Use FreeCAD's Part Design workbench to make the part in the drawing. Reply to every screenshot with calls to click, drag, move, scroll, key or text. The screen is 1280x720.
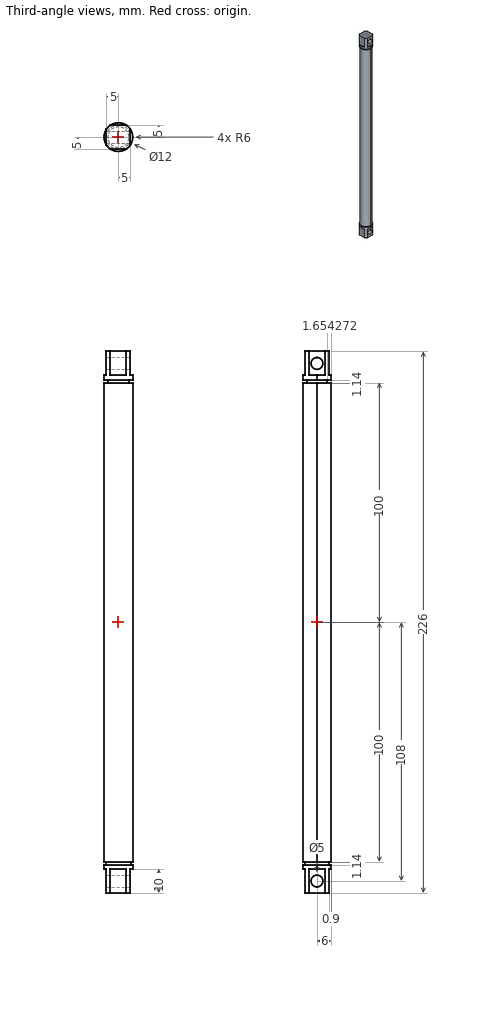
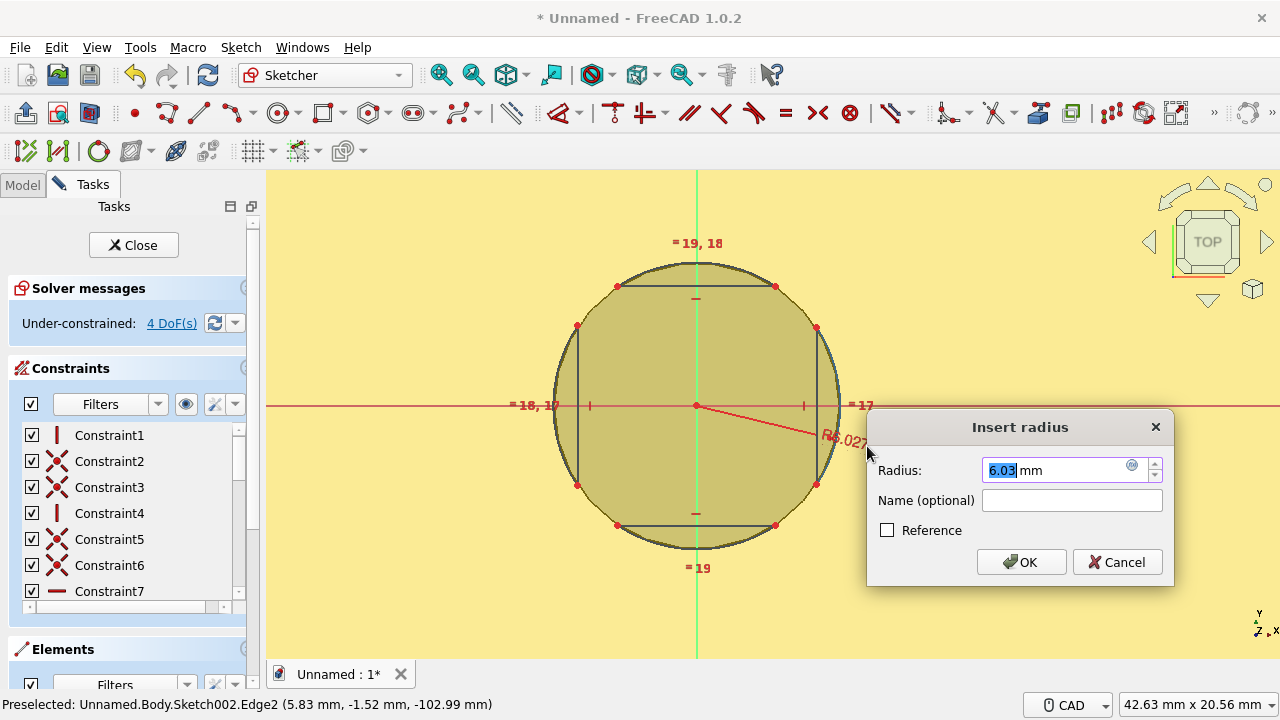
text(6)
key(Return)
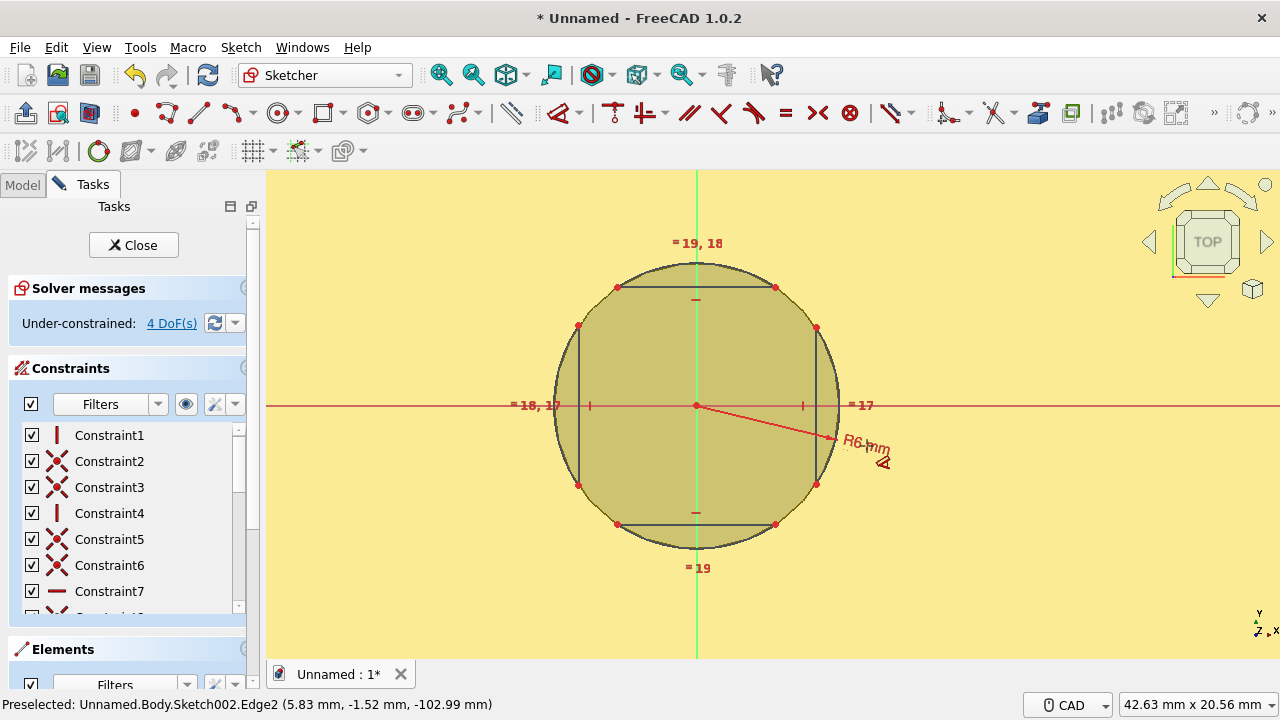
click(816, 484)
click(798, 518)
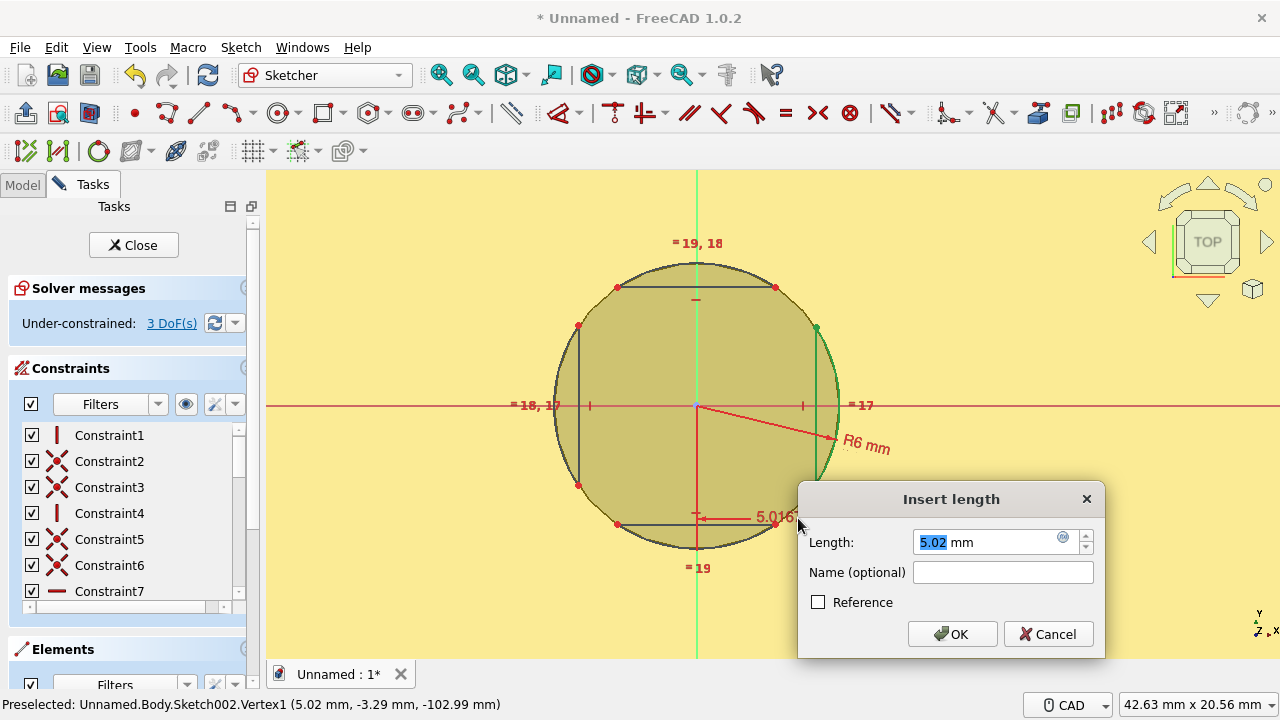
text(5)
key(Return)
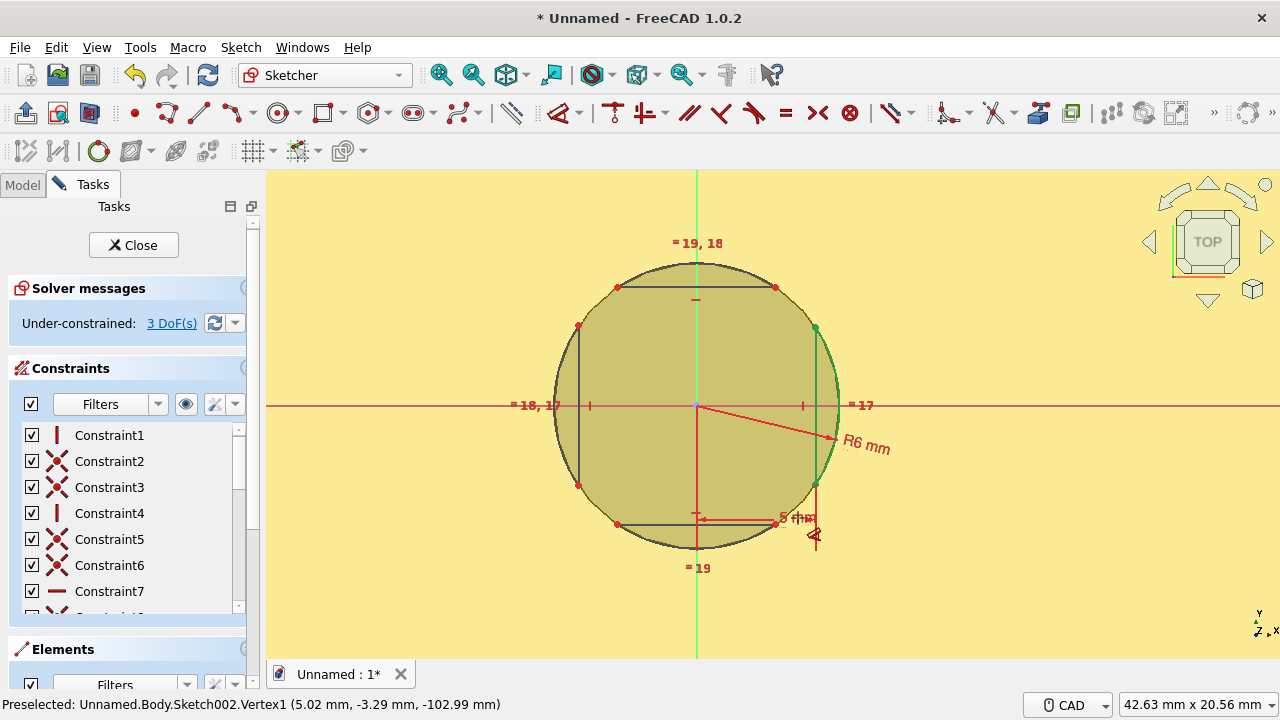
click(579, 326)
click(596, 292)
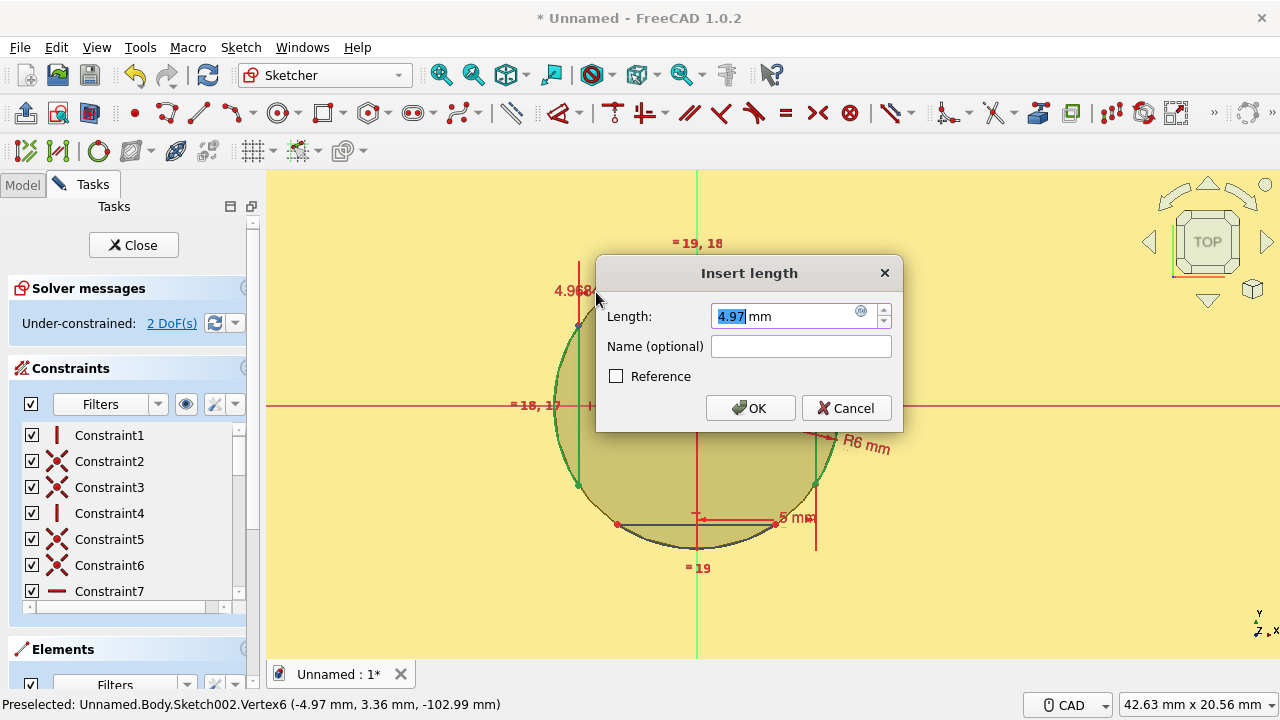
text(5)
key(Return)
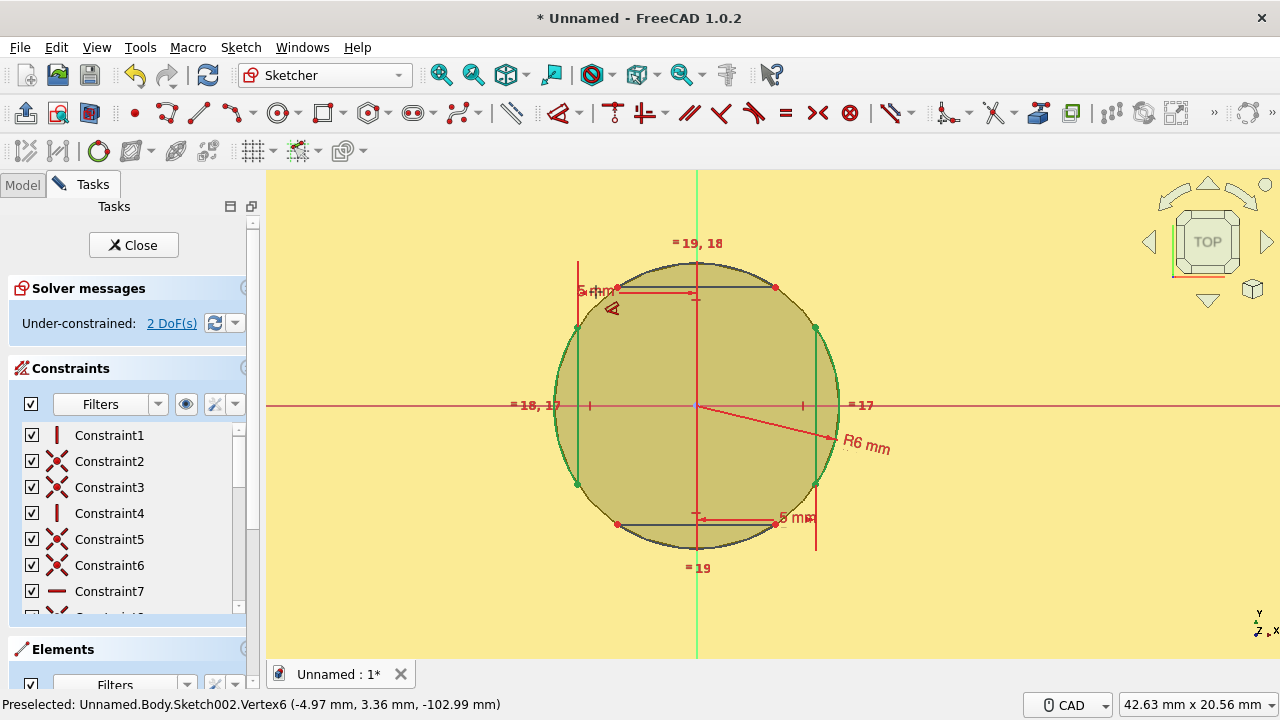
click(776, 287)
click(810, 305)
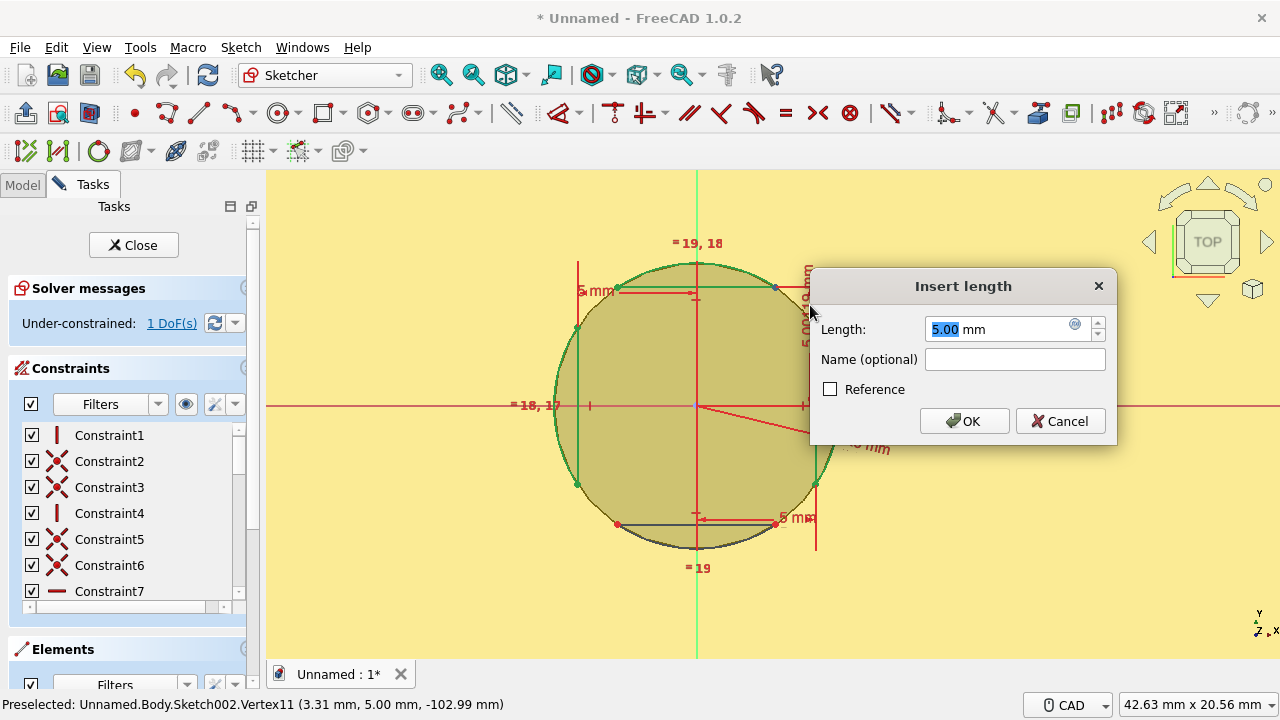
text(5)
key(Return)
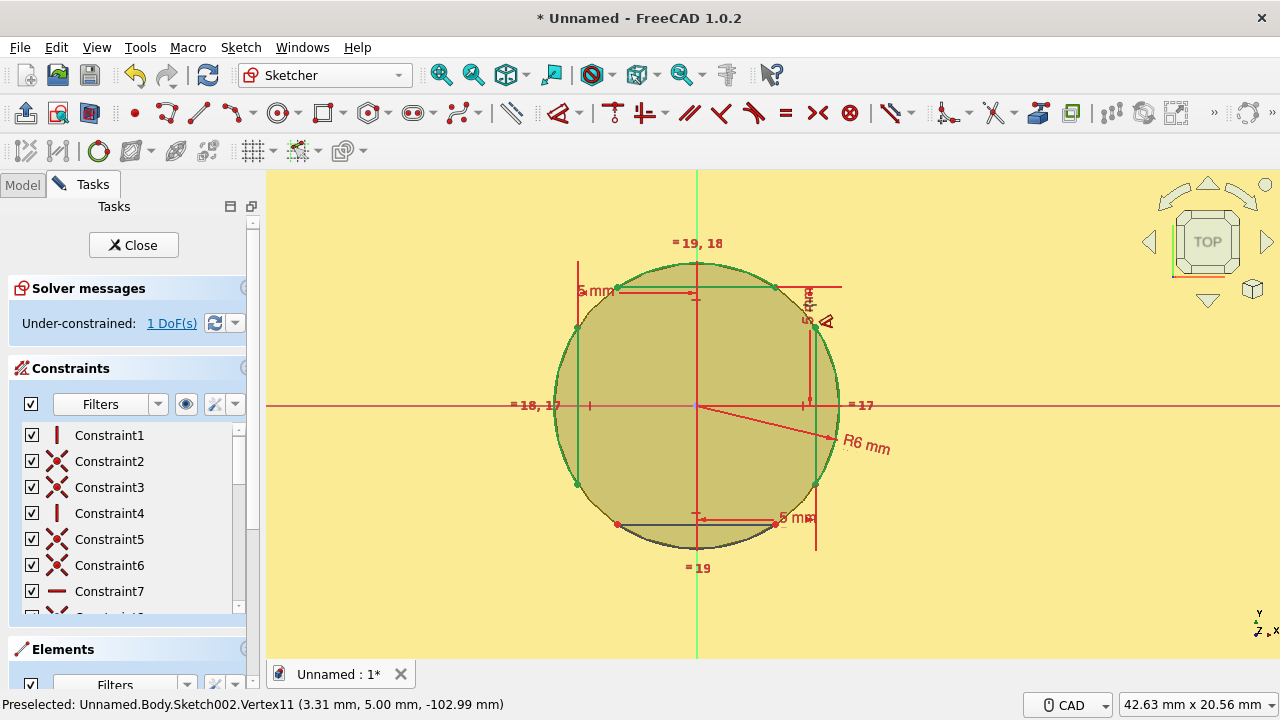
click(618, 525)
click(584, 507)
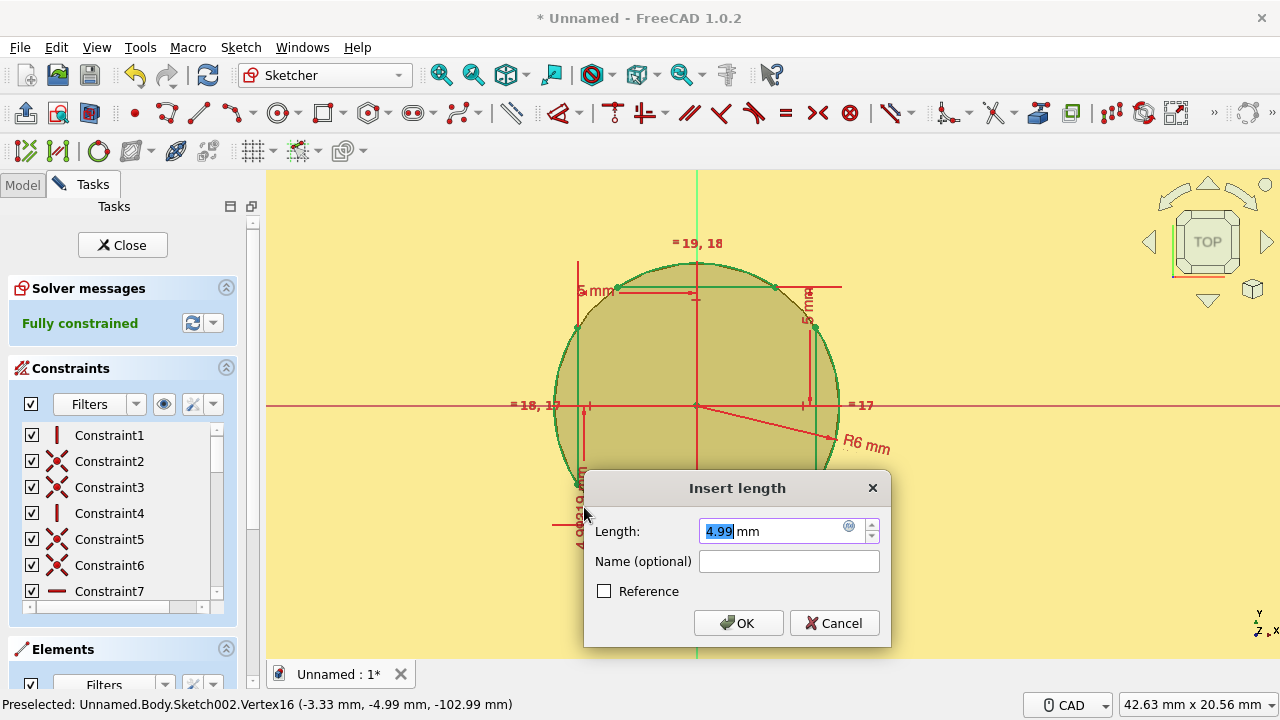
text(5)
key(Return)
key(Escape)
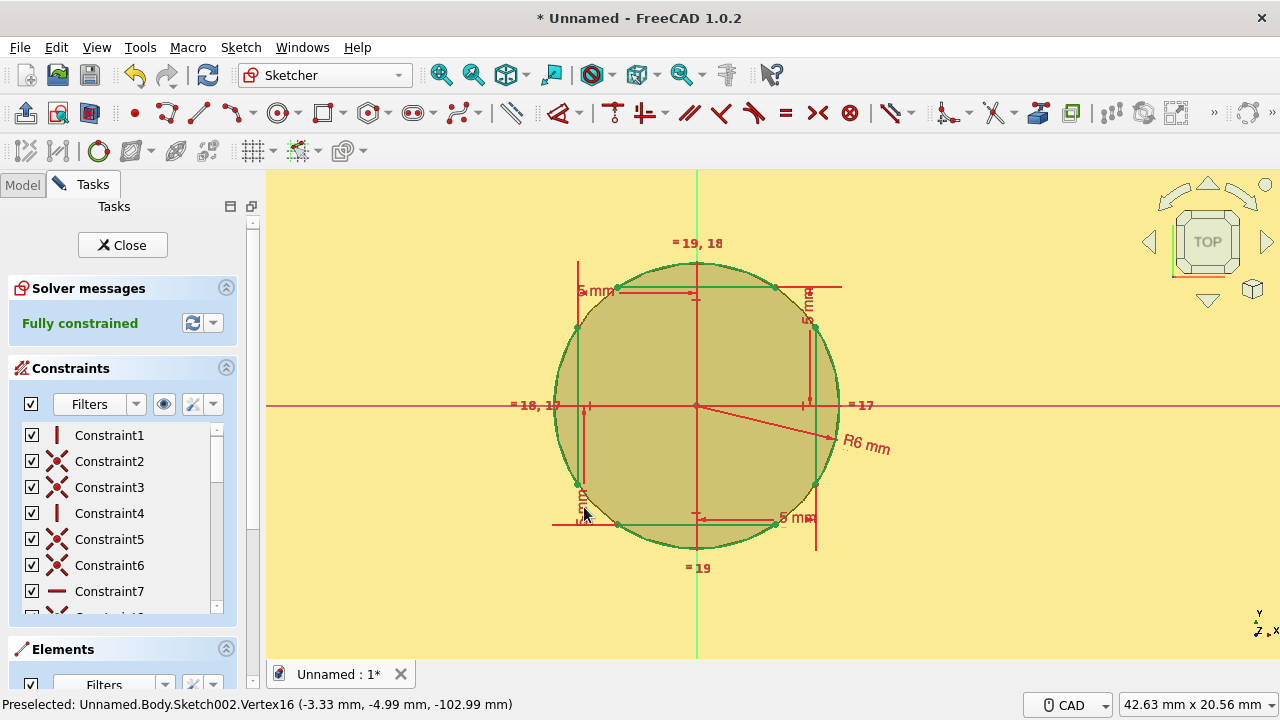
click(123, 245)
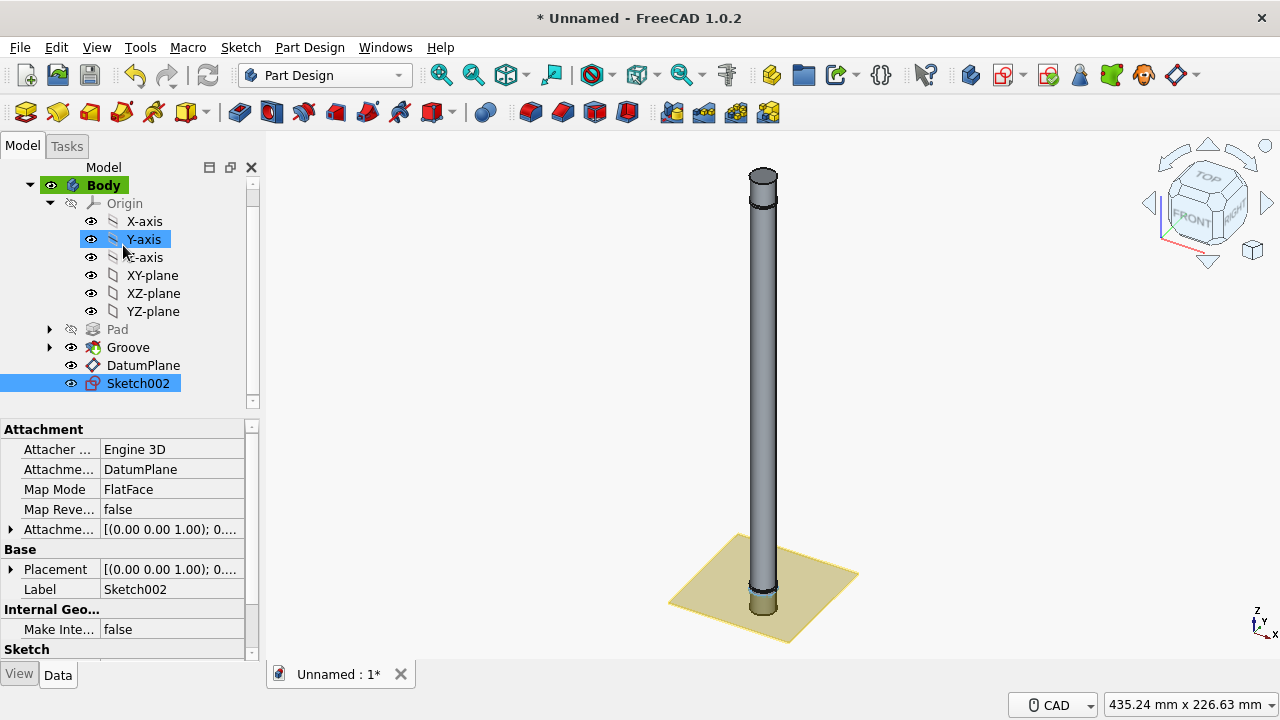
click(240, 112)